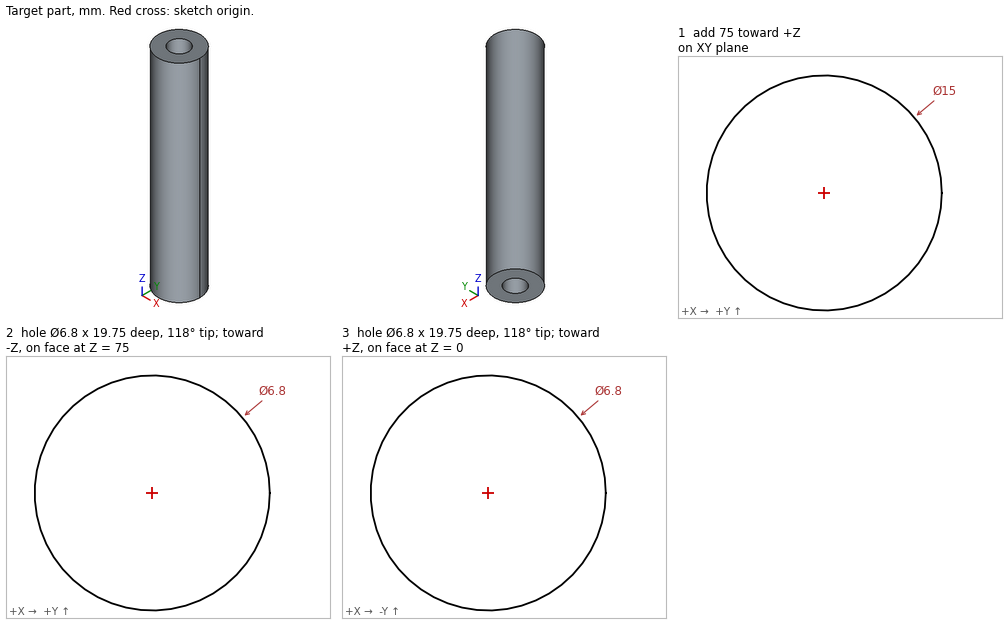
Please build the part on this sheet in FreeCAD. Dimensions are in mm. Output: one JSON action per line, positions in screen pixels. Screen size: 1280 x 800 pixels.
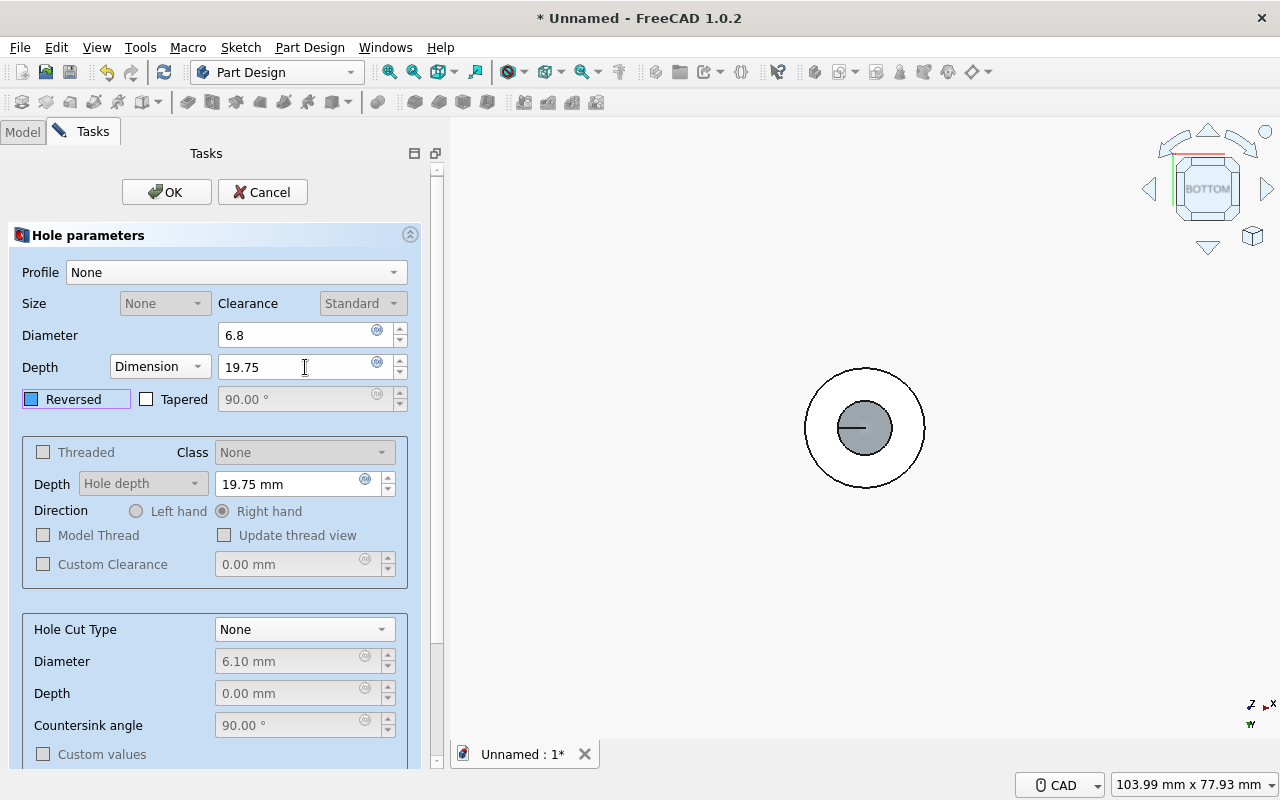
{"action": "left_click", "coordinate": [167, 192]}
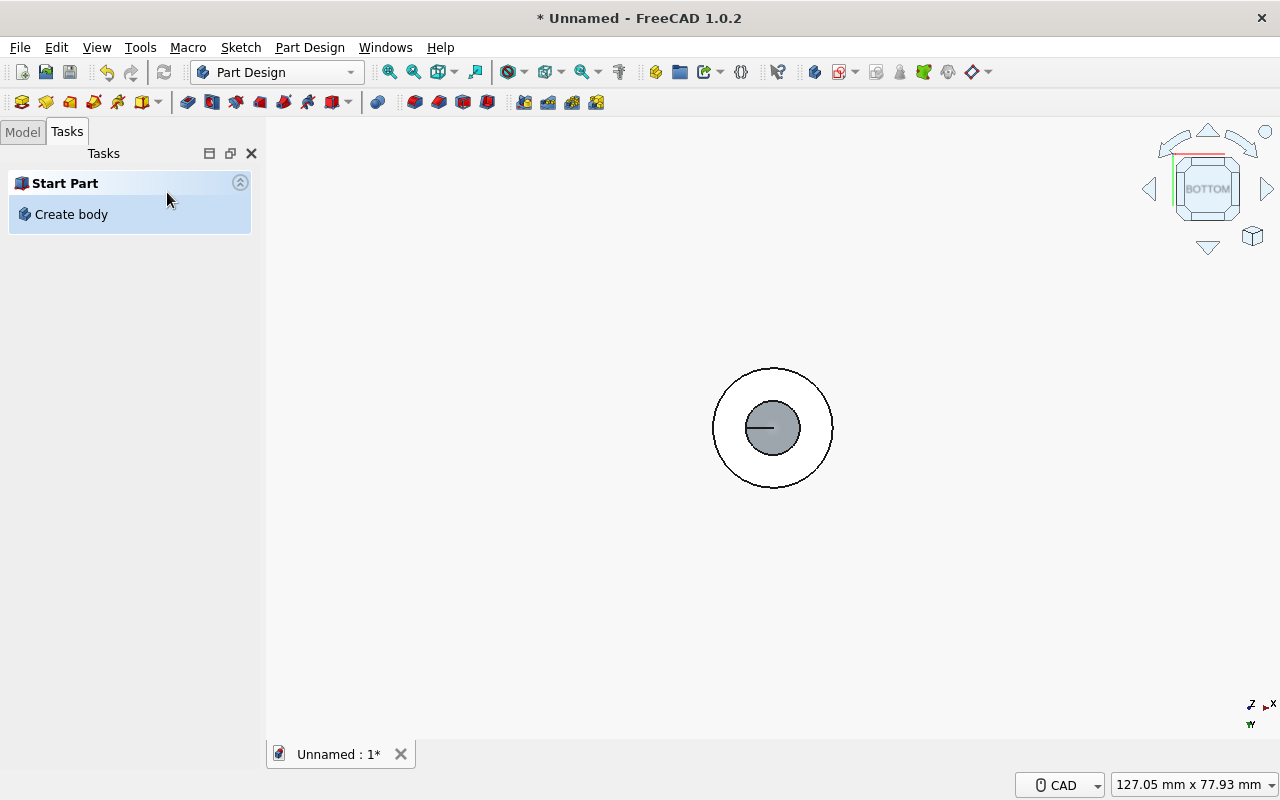
{"action": "key", "text": "0"}